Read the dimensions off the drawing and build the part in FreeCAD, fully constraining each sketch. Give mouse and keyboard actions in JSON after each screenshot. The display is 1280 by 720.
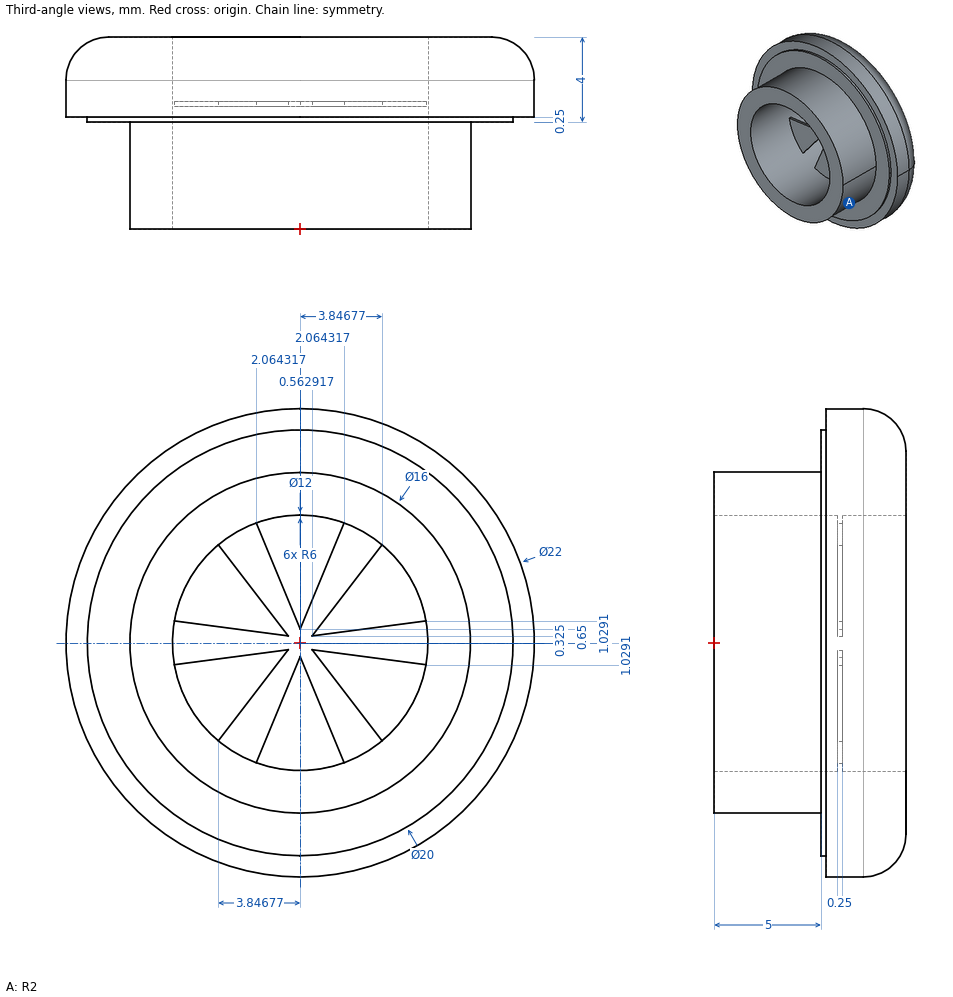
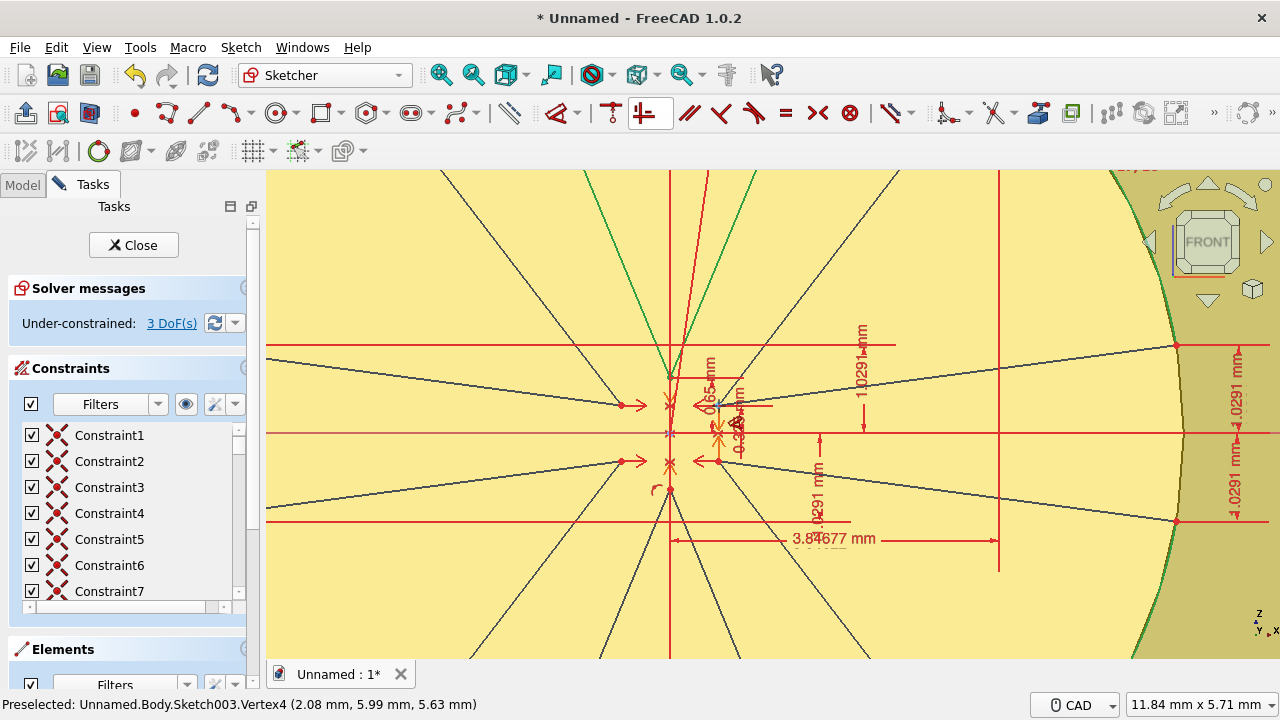
{"action": "left_click", "coordinate": [719, 406]}
{"action": "left_click", "coordinate": [694, 467]}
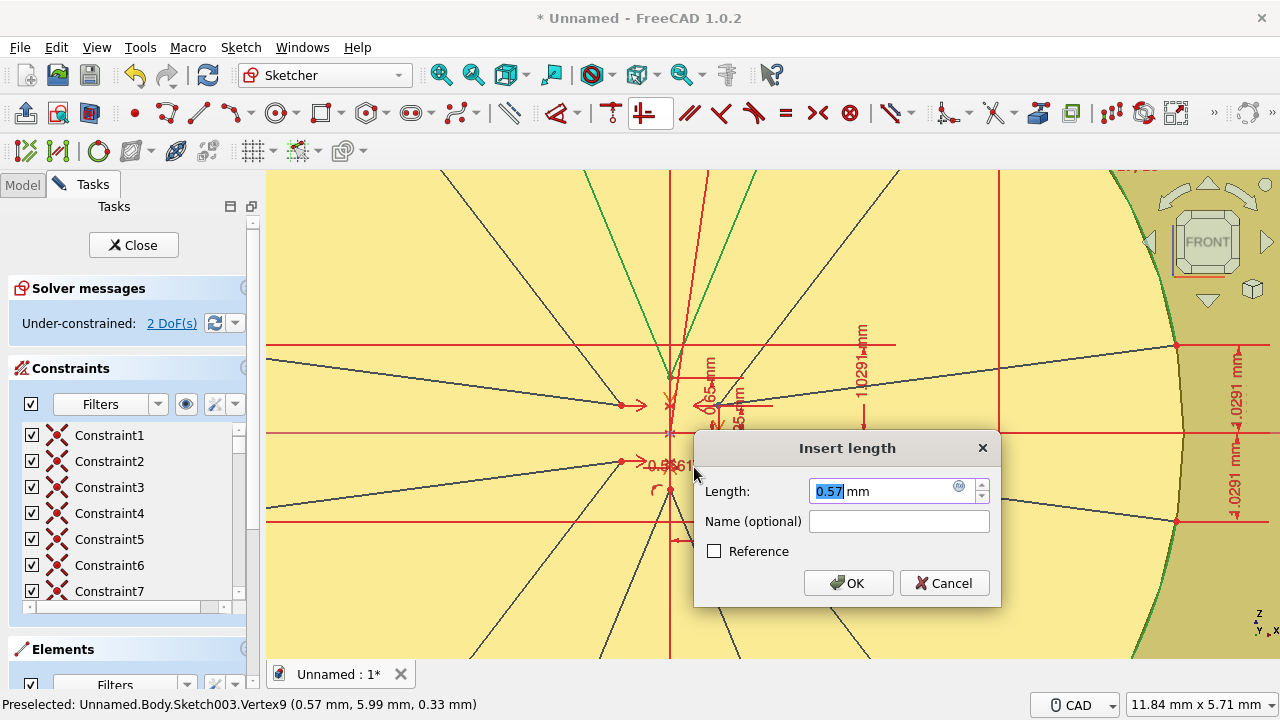
{"action": "type", "text": "0.562917"}
{"action": "key", "text": "Return"}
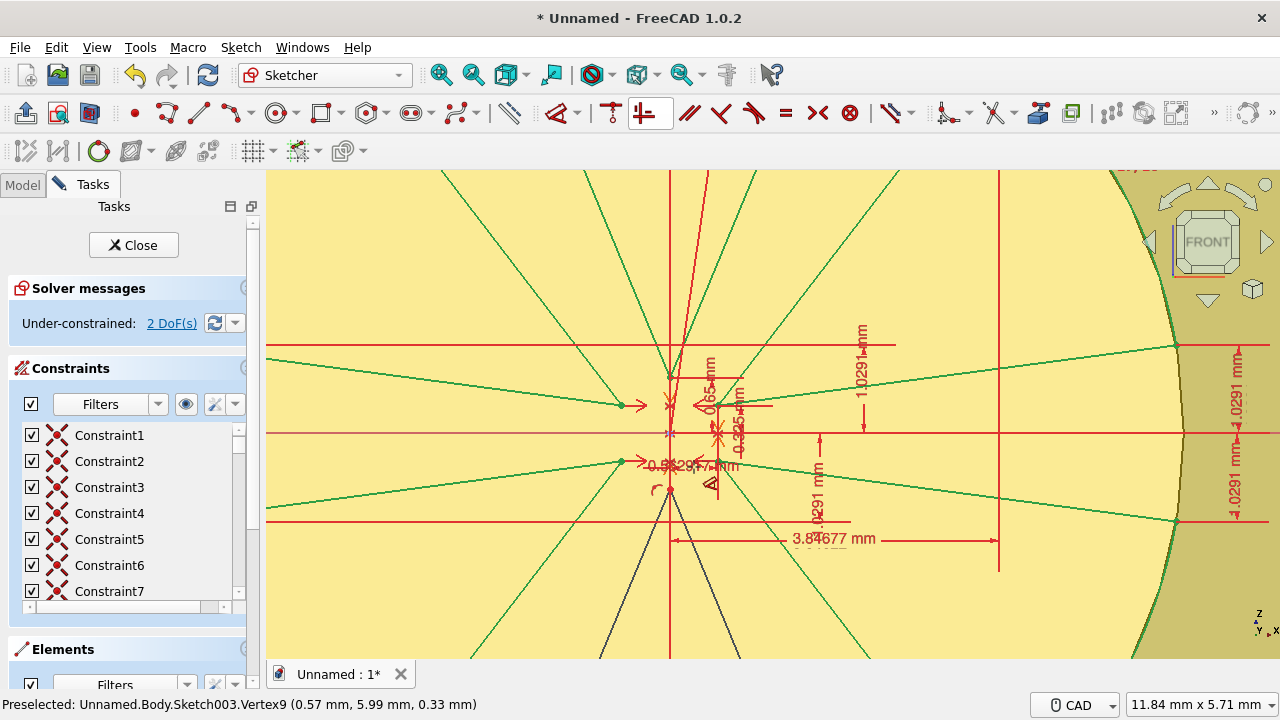
{"action": "scroll", "coordinate": [719, 406], "scroll_direction": "down", "scroll_amount": 6}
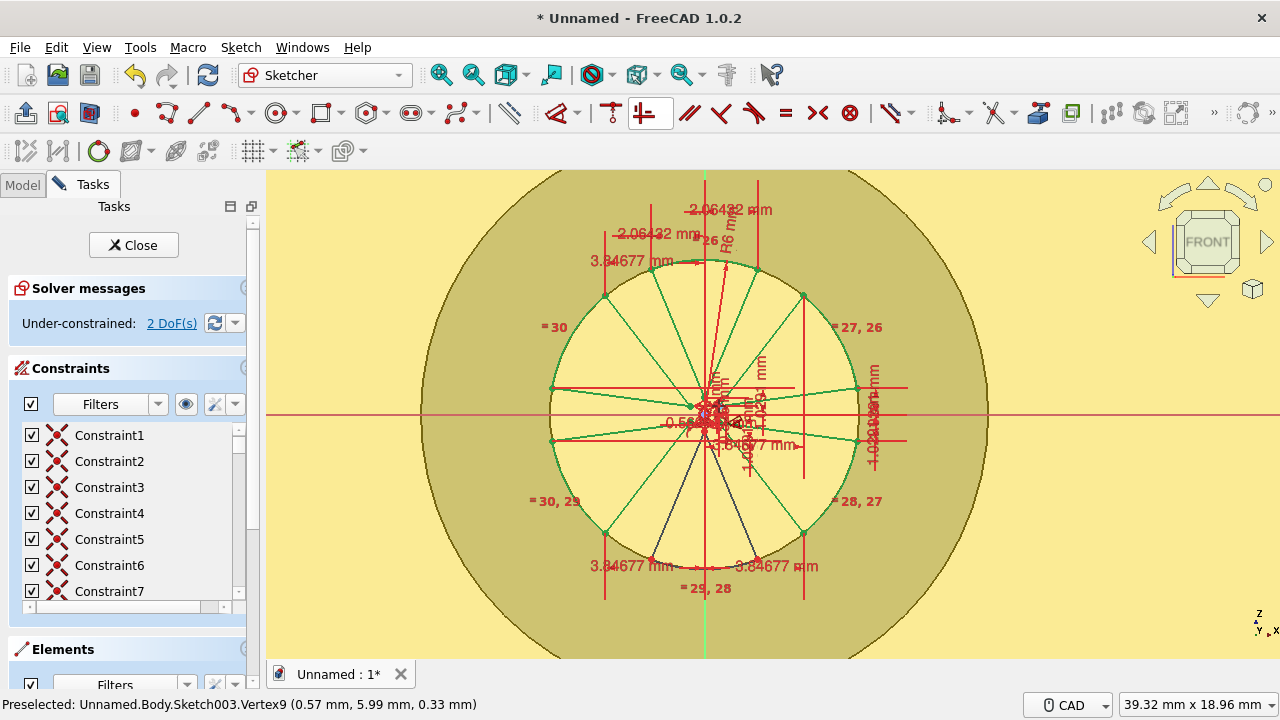
{"action": "left_click", "coordinate": [758, 560]}
{"action": "left_click", "coordinate": [731, 594]}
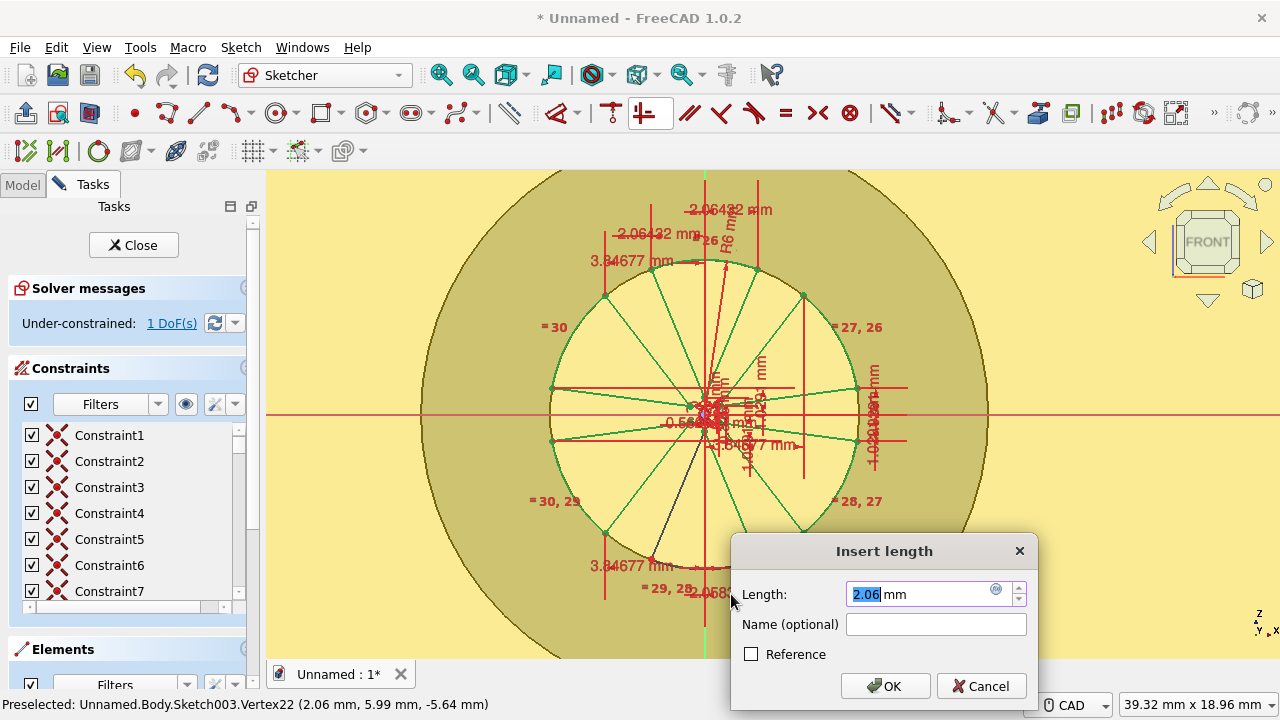
{"action": "type", "text": "2.064317"}
{"action": "key", "text": "Return"}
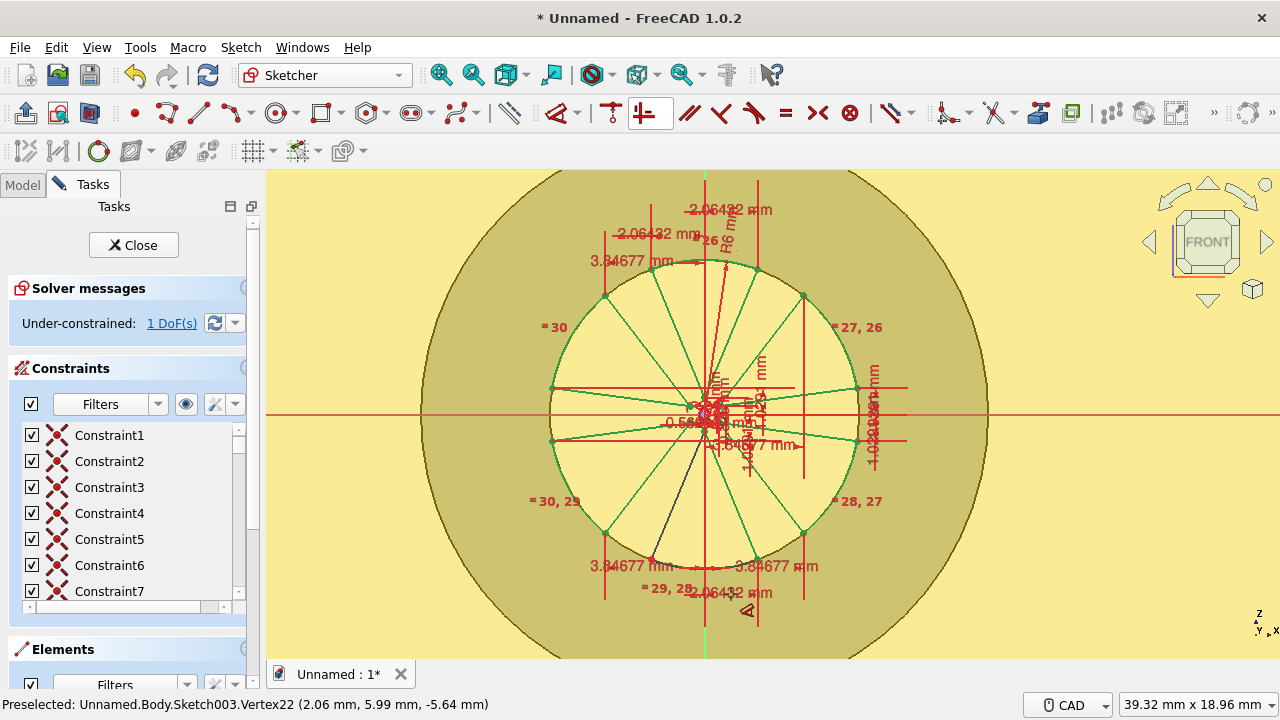
{"action": "left_click", "coordinate": [651, 560]}
{"action": "left_click", "coordinate": [659, 594]}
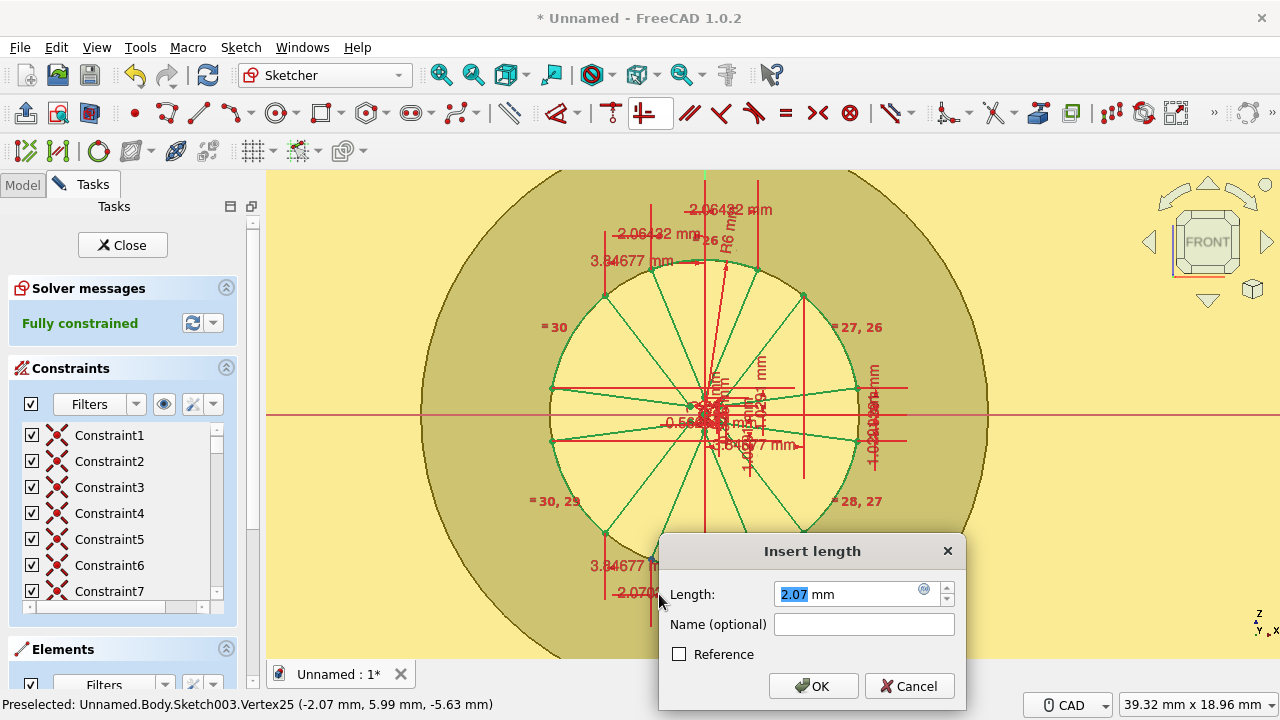
{"action": "type", "text": "2.064317"}
{"action": "key", "text": "Return"}
{"action": "key", "text": "Escape"}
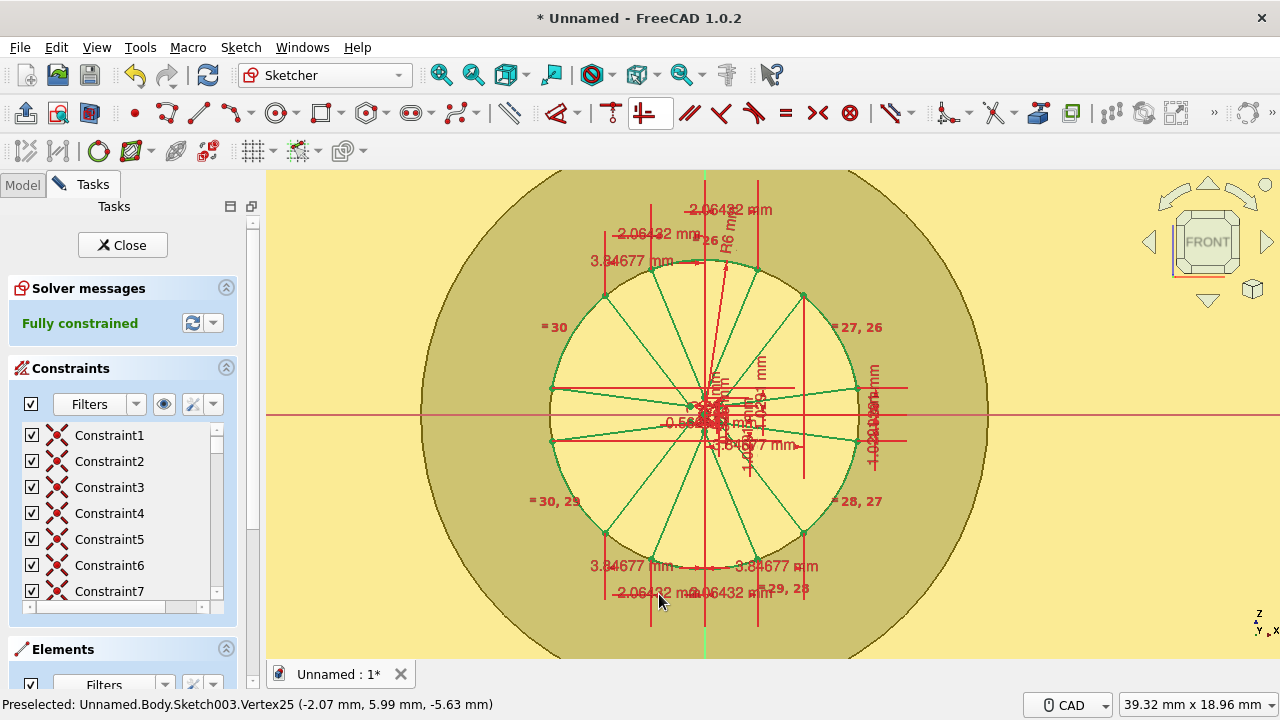
{"action": "left_click", "coordinate": [123, 245]}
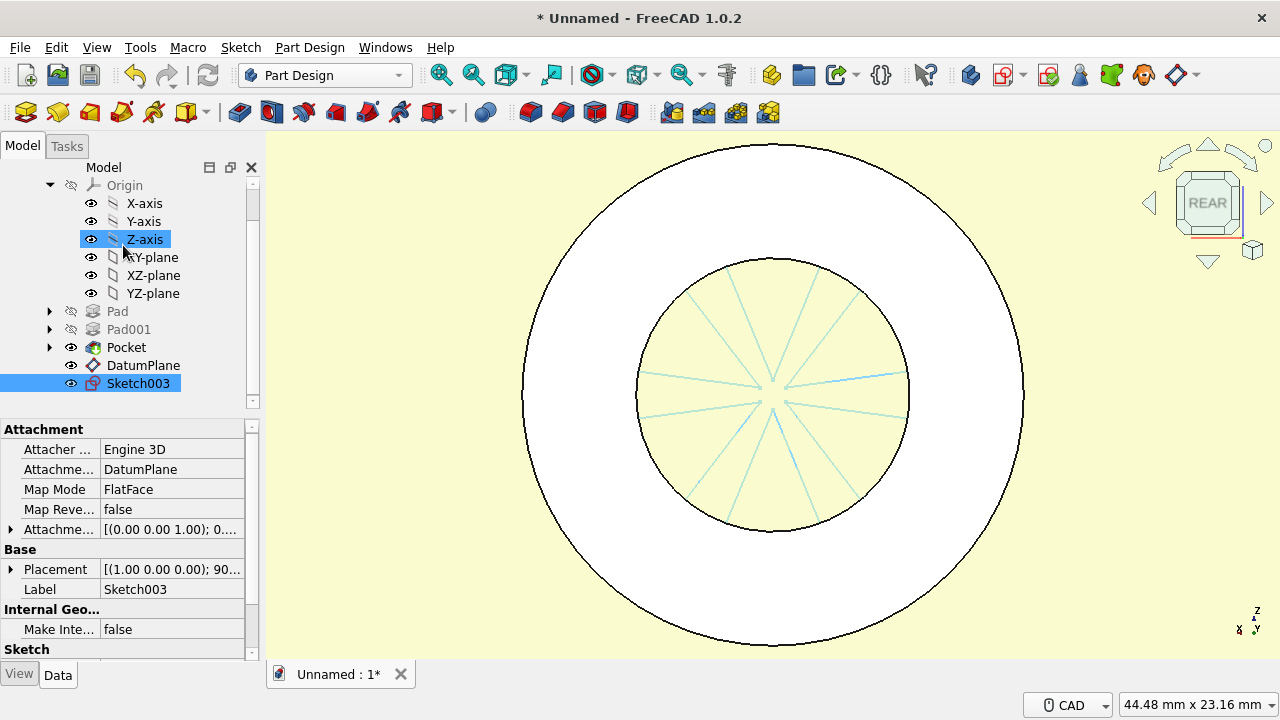
{"action": "left_click", "coordinate": [26, 112]}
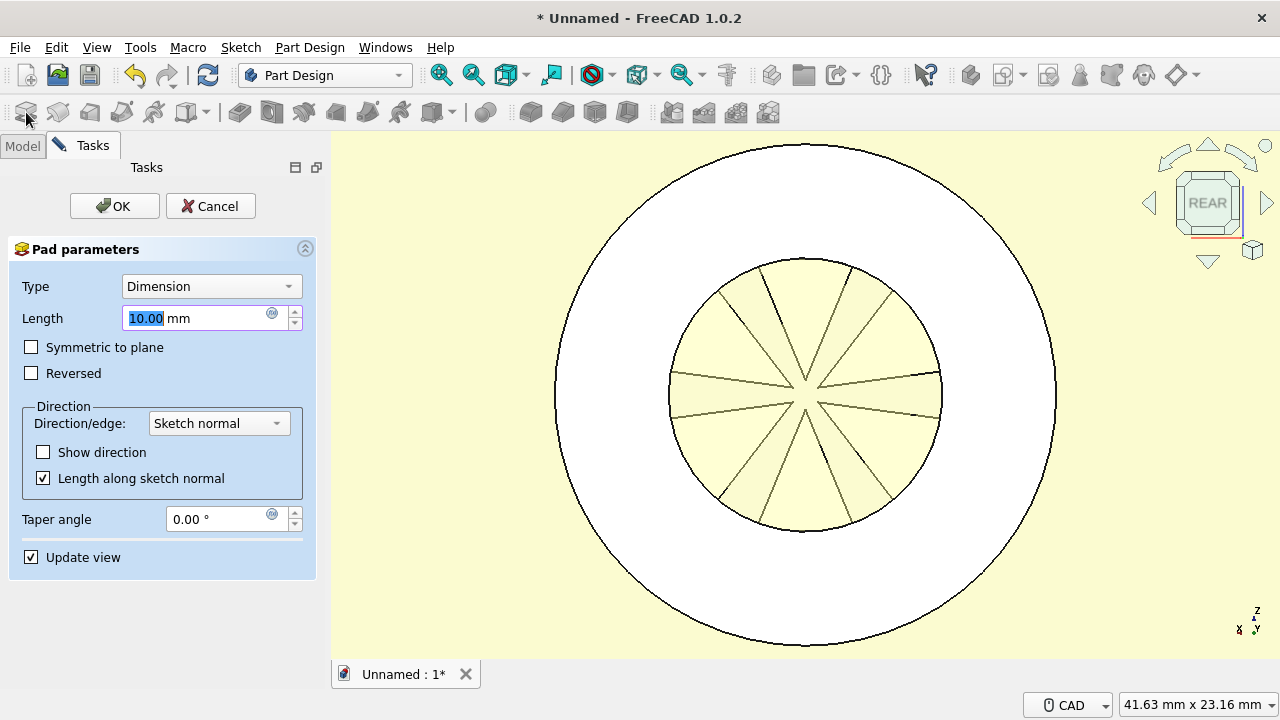
{"action": "type", "text": "0.25"}
{"action": "key", "text": "Tab"}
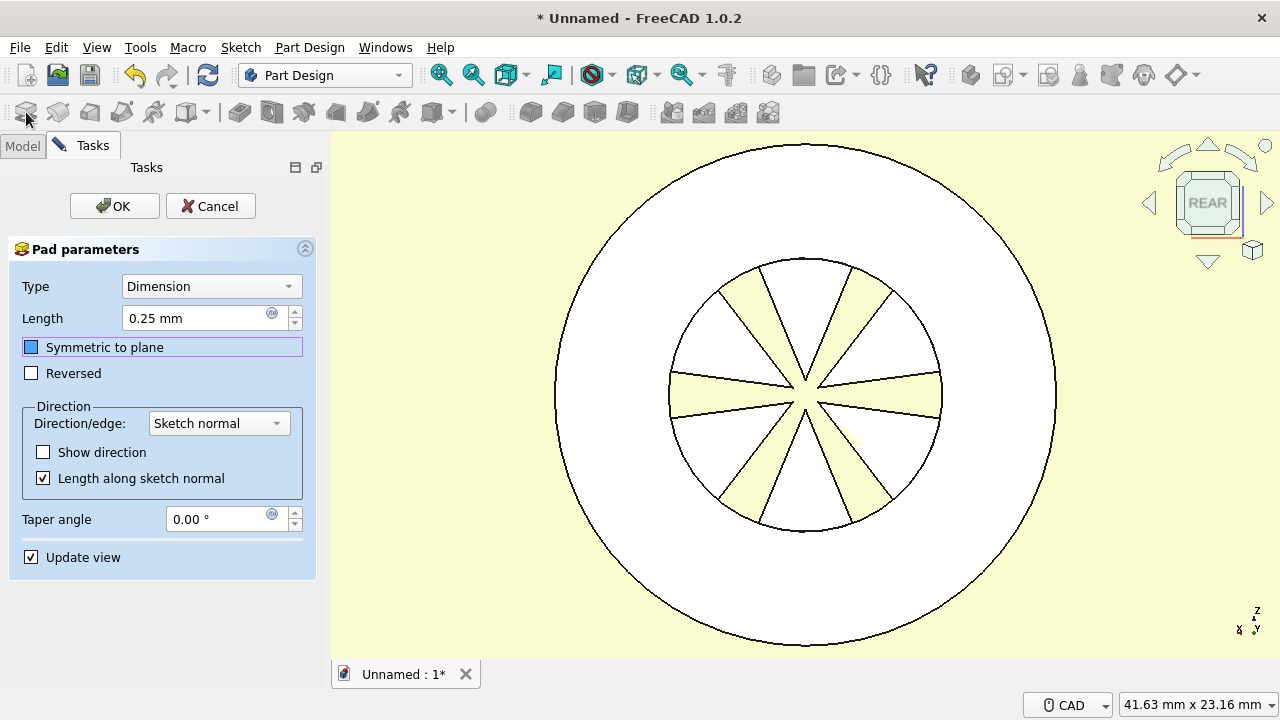
{"action": "left_click", "coordinate": [115, 206]}